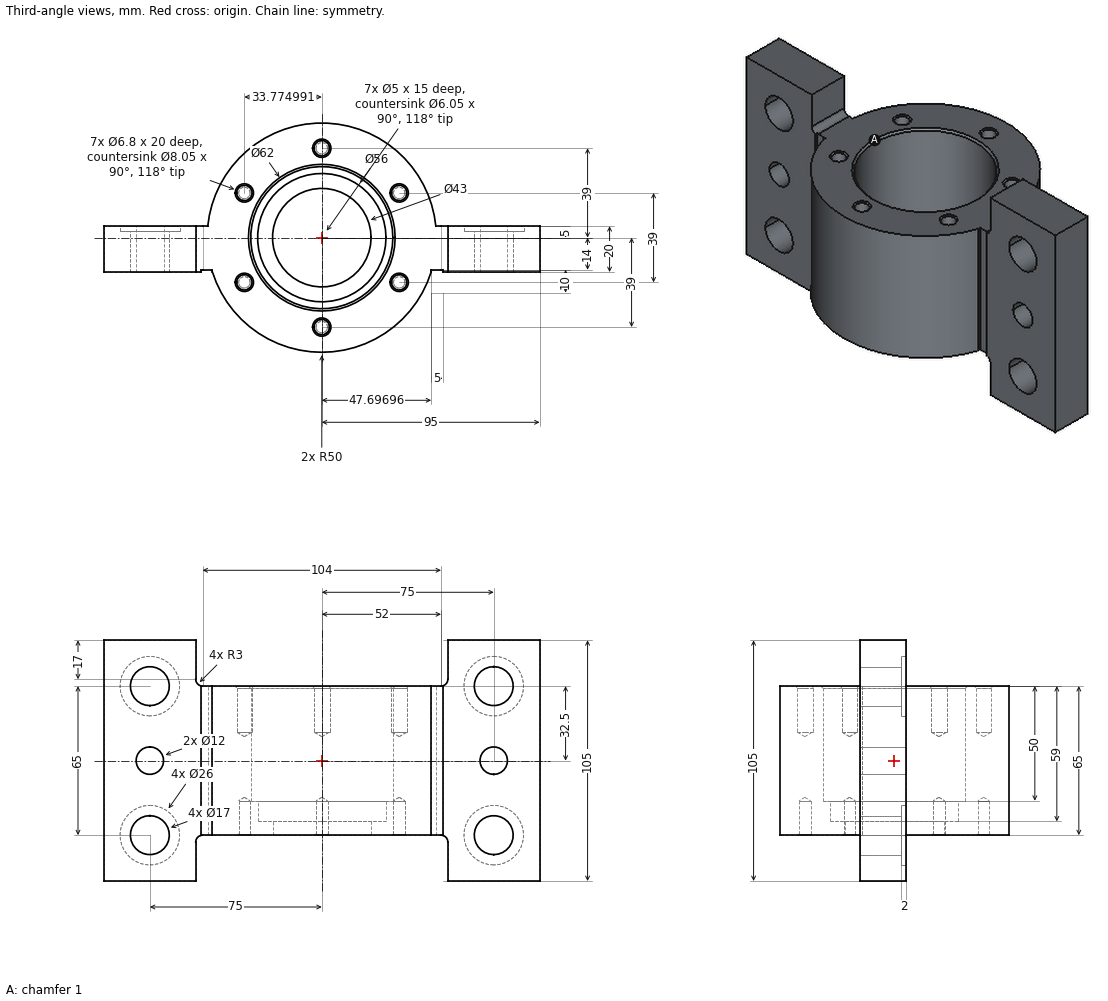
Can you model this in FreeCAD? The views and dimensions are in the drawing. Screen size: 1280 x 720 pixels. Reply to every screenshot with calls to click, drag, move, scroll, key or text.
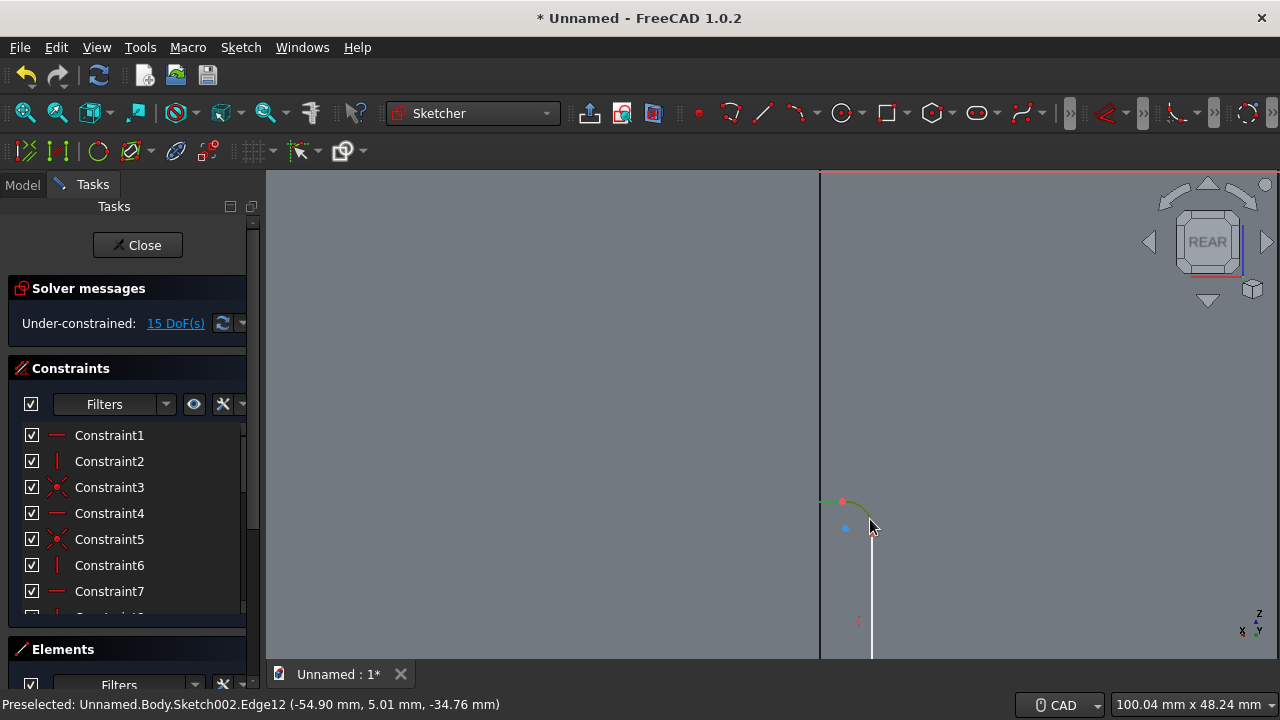
key(t)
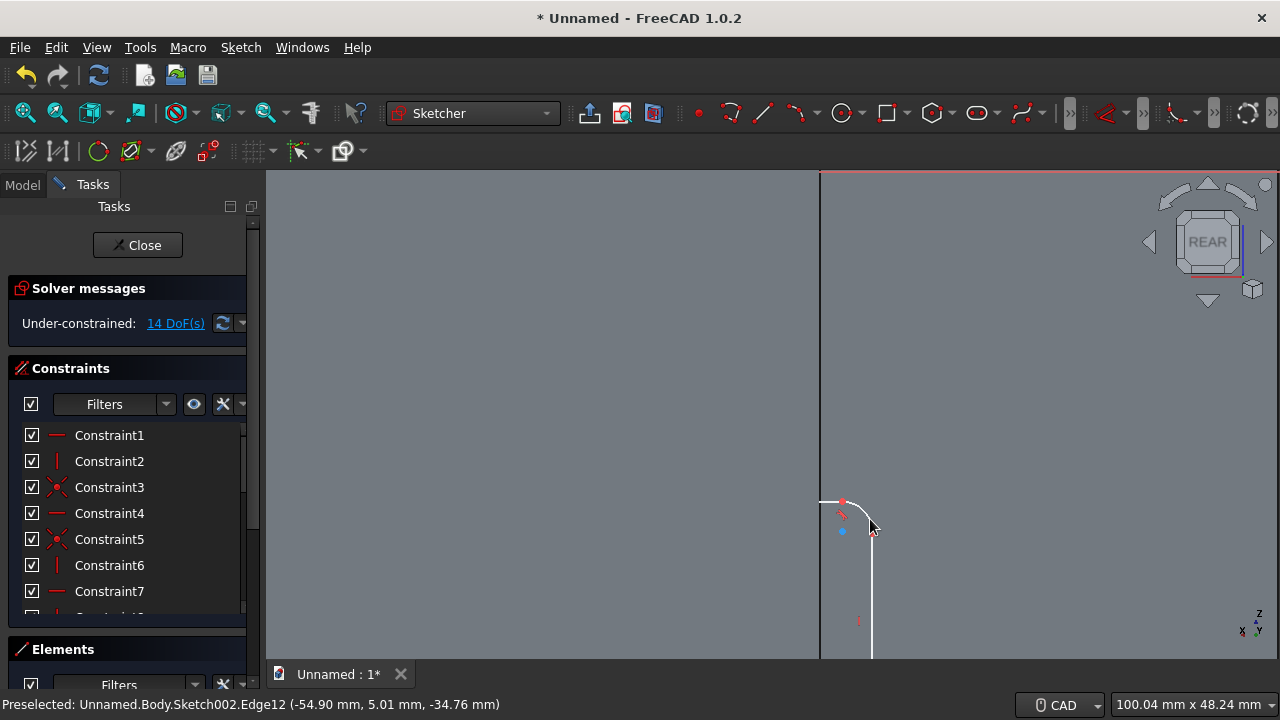
scroll(872, 519, down, 6)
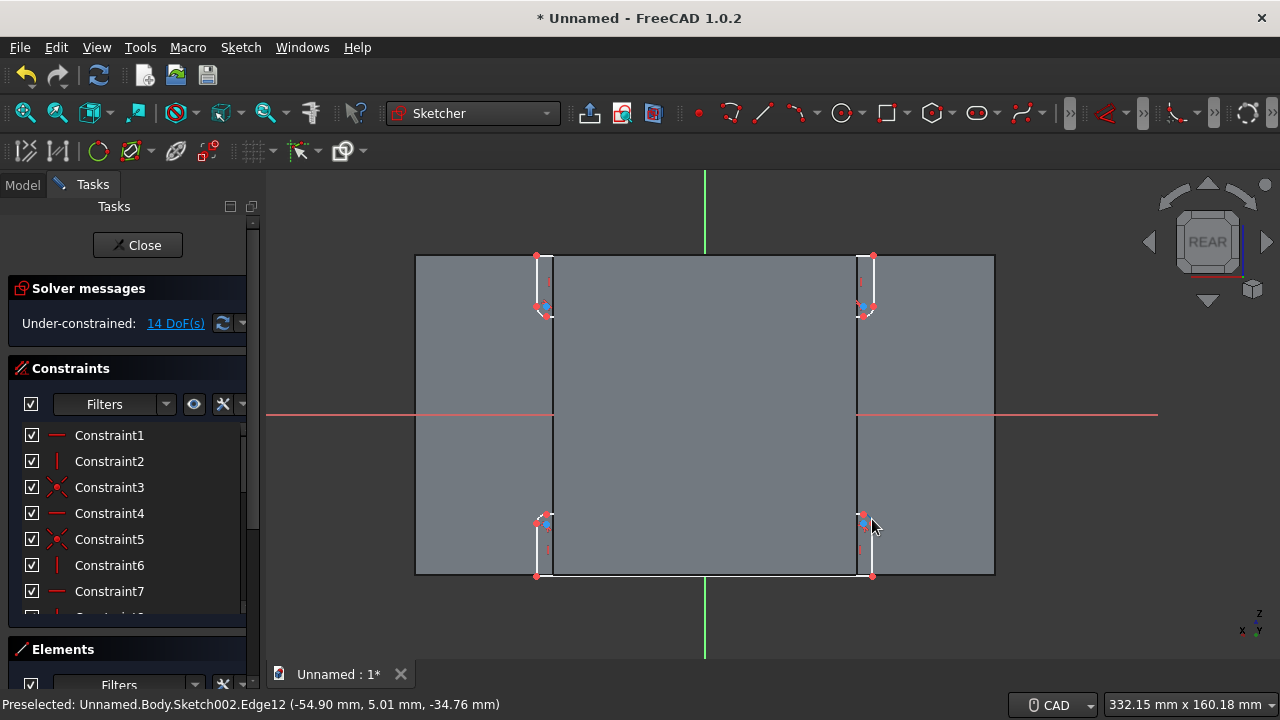
click(537, 540)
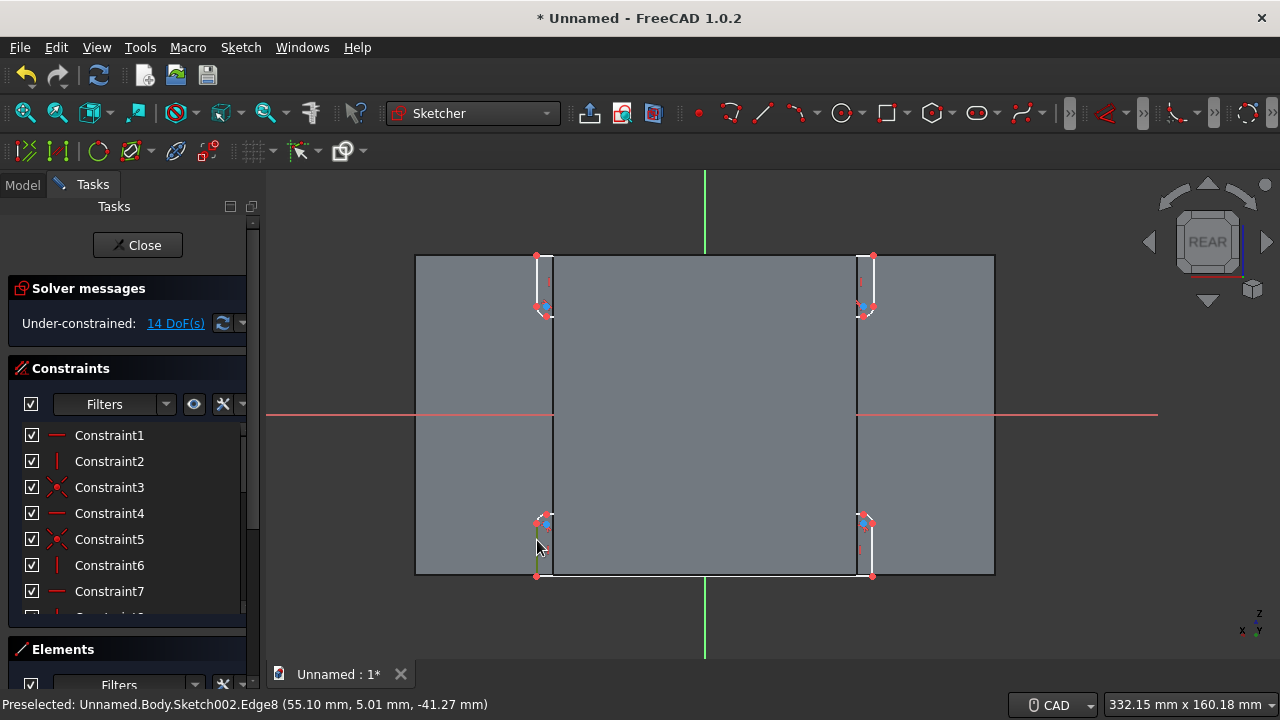
scroll(540, 517, up, 4)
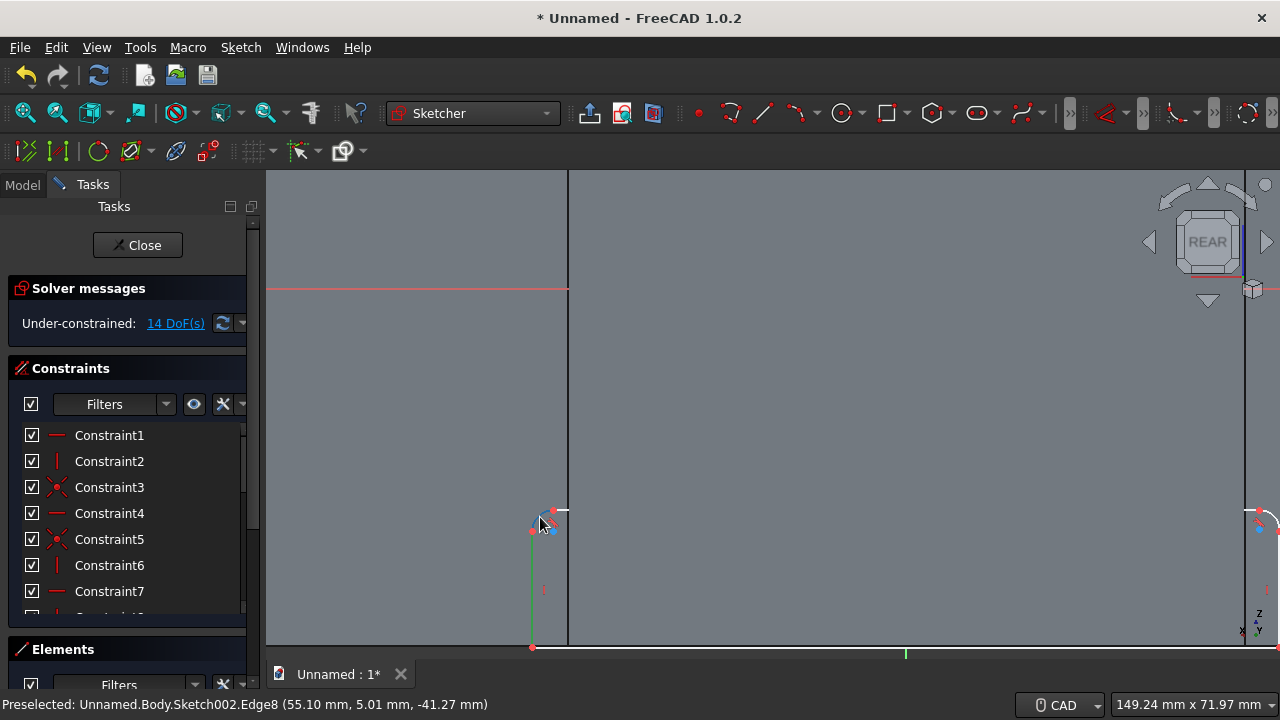
click(539, 516)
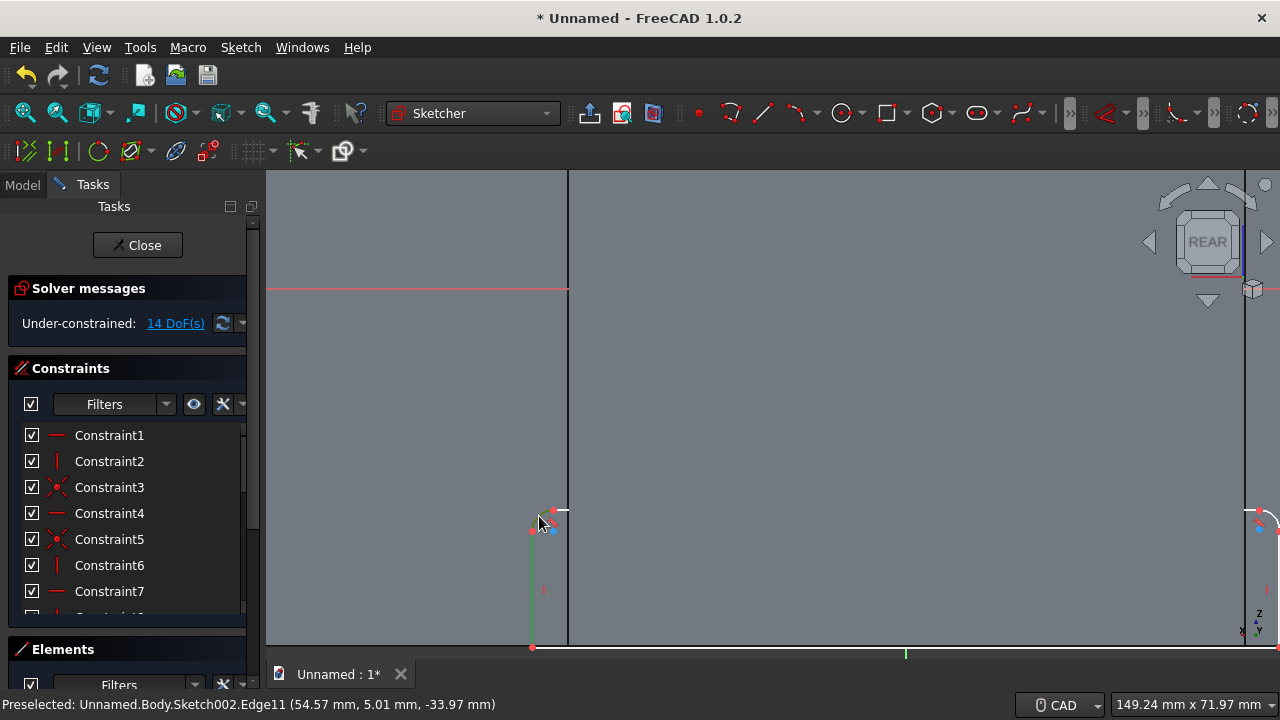
key(t)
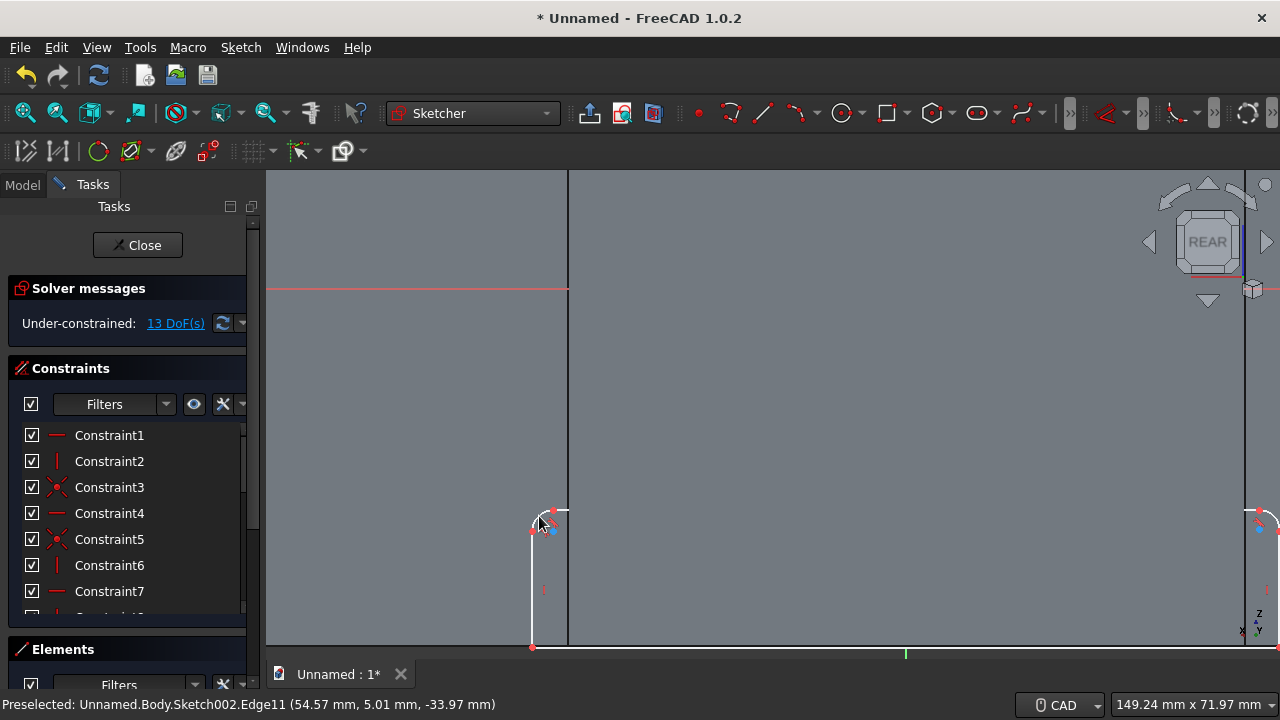
scroll(540, 517, down, 4)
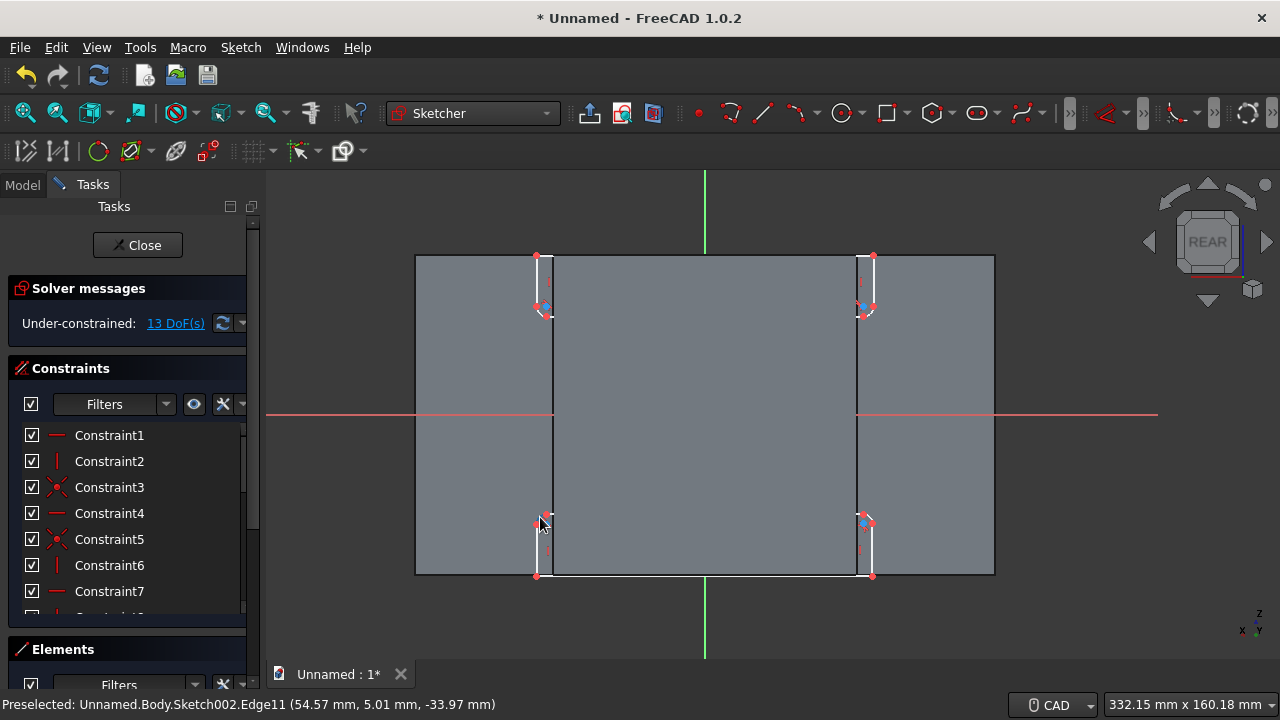
click(872, 560)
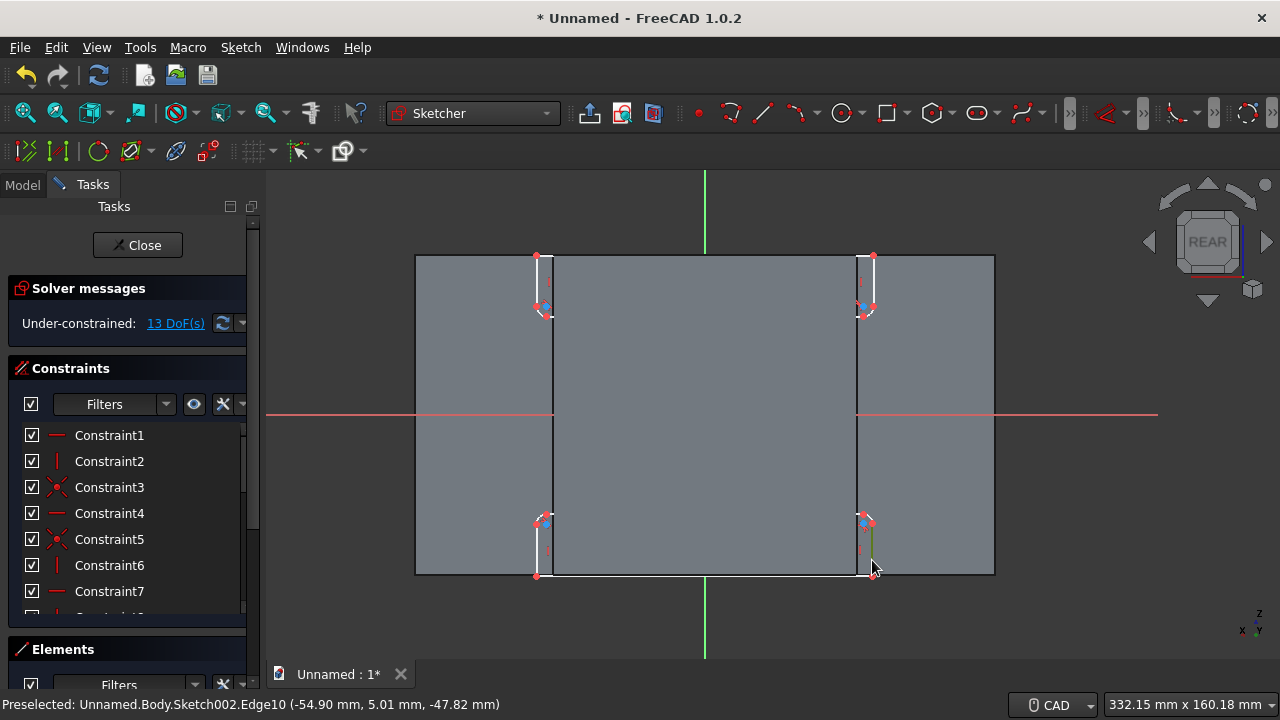
scroll(870, 517, up, 4)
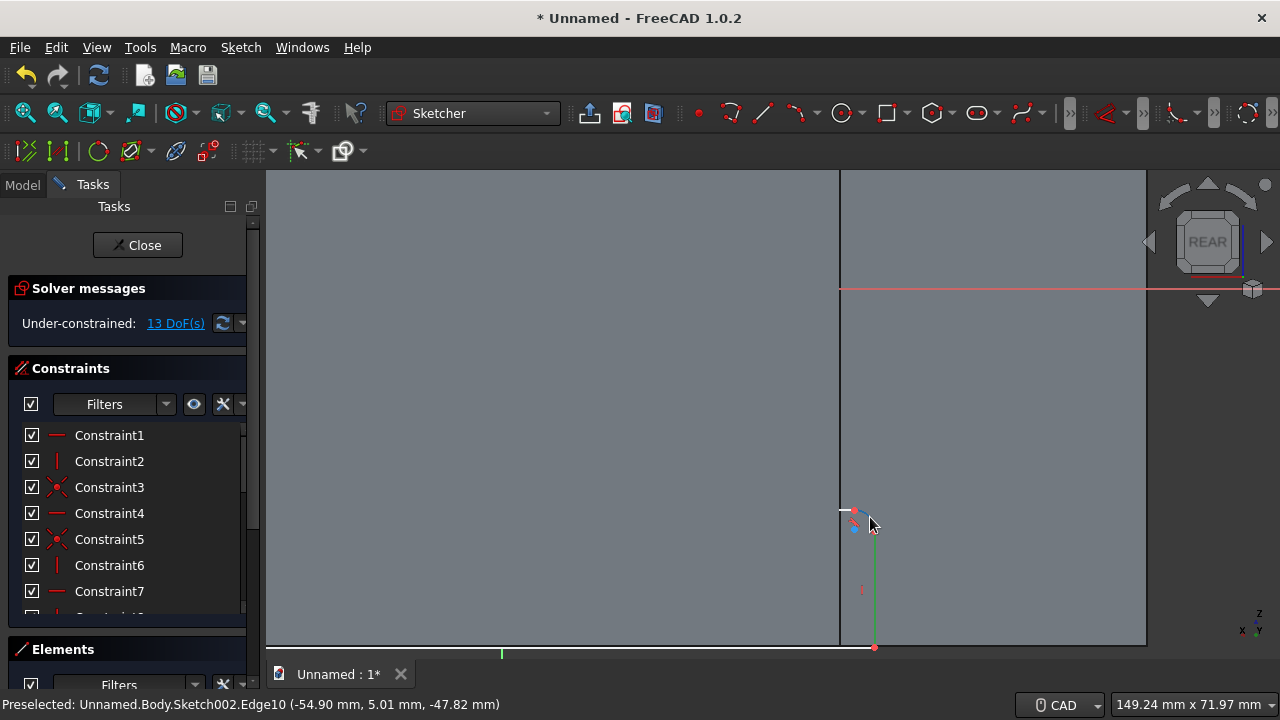
click(869, 516)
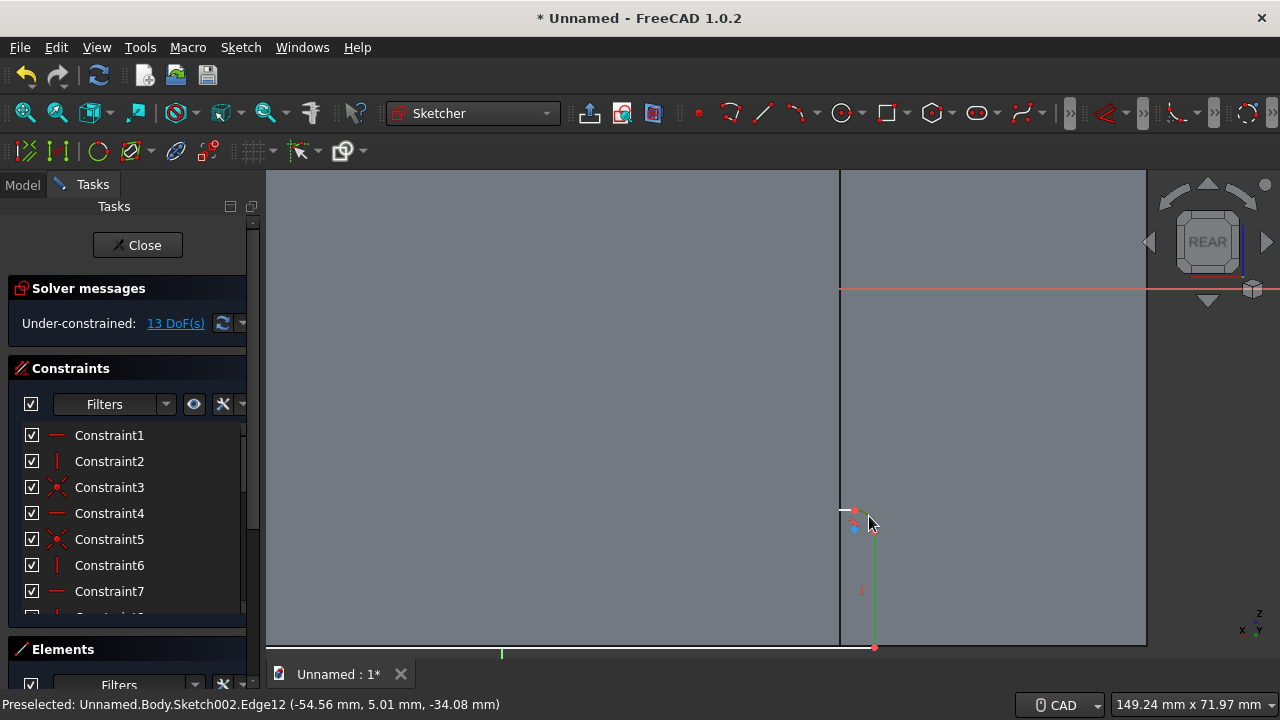
key(t)